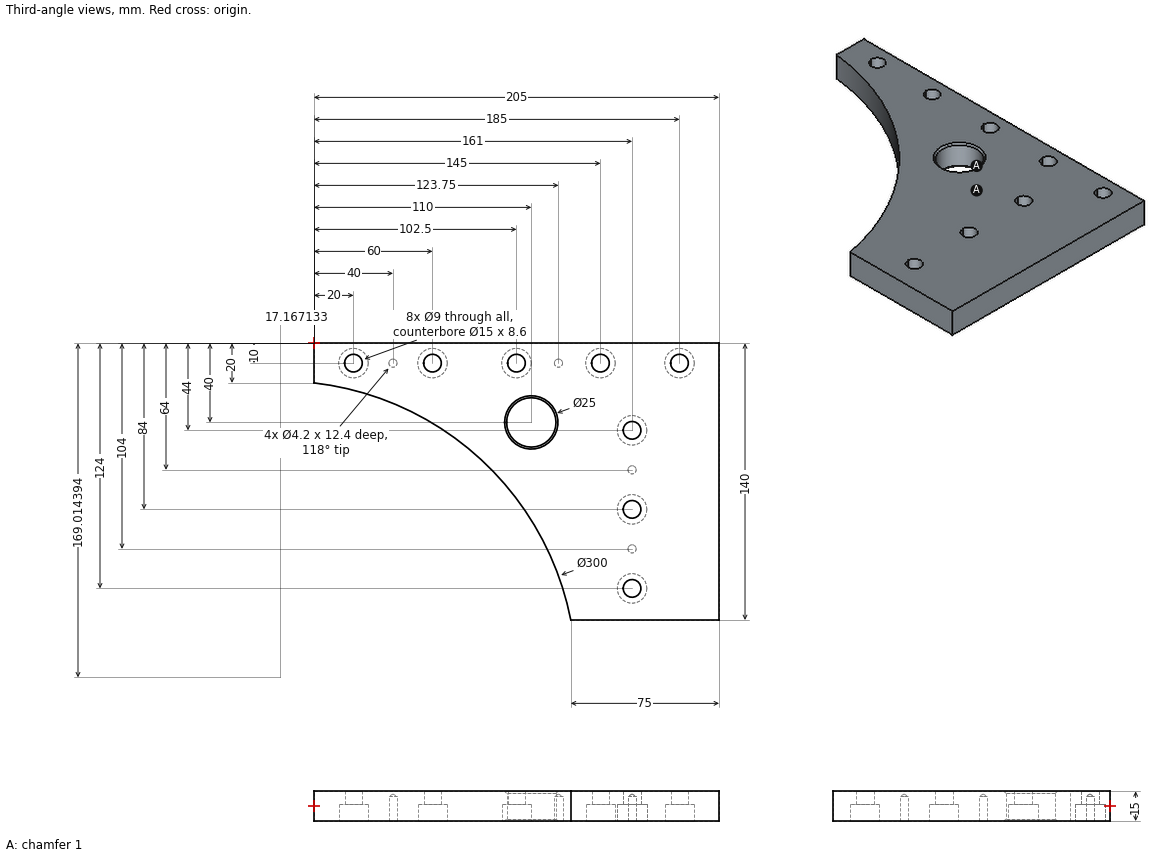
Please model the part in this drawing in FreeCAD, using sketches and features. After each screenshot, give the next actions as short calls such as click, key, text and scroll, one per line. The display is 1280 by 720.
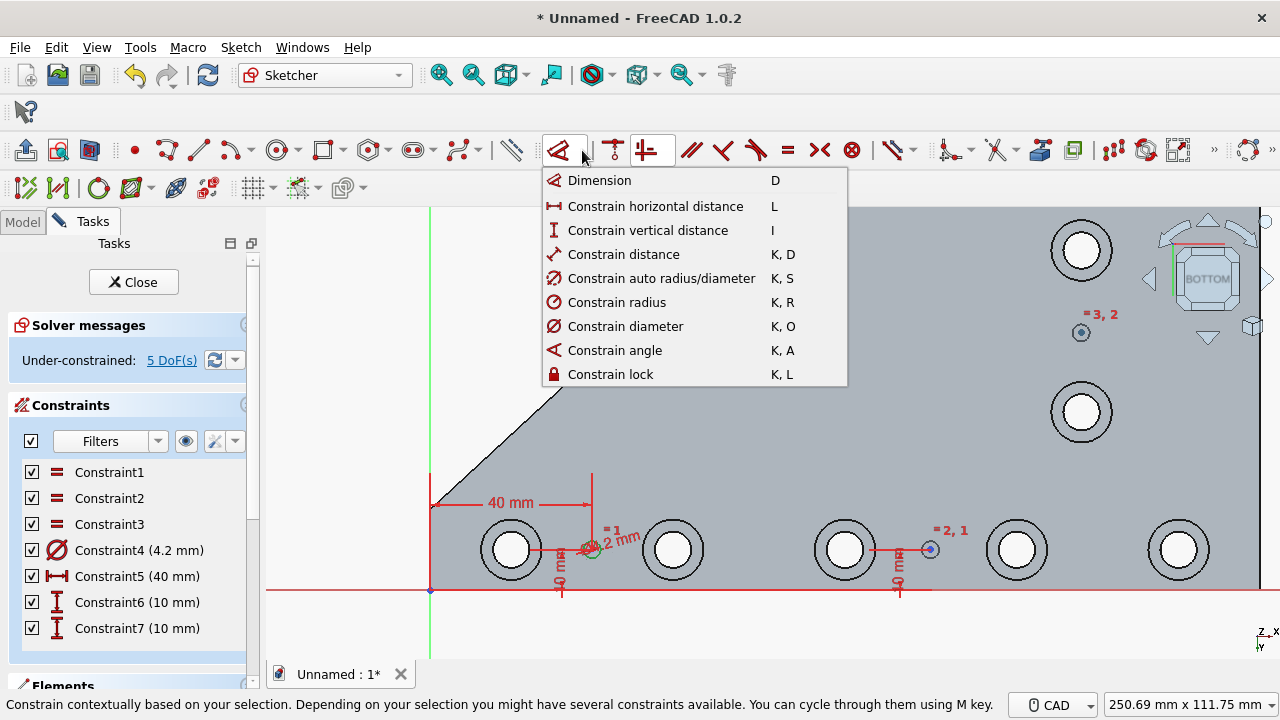
click(695, 230)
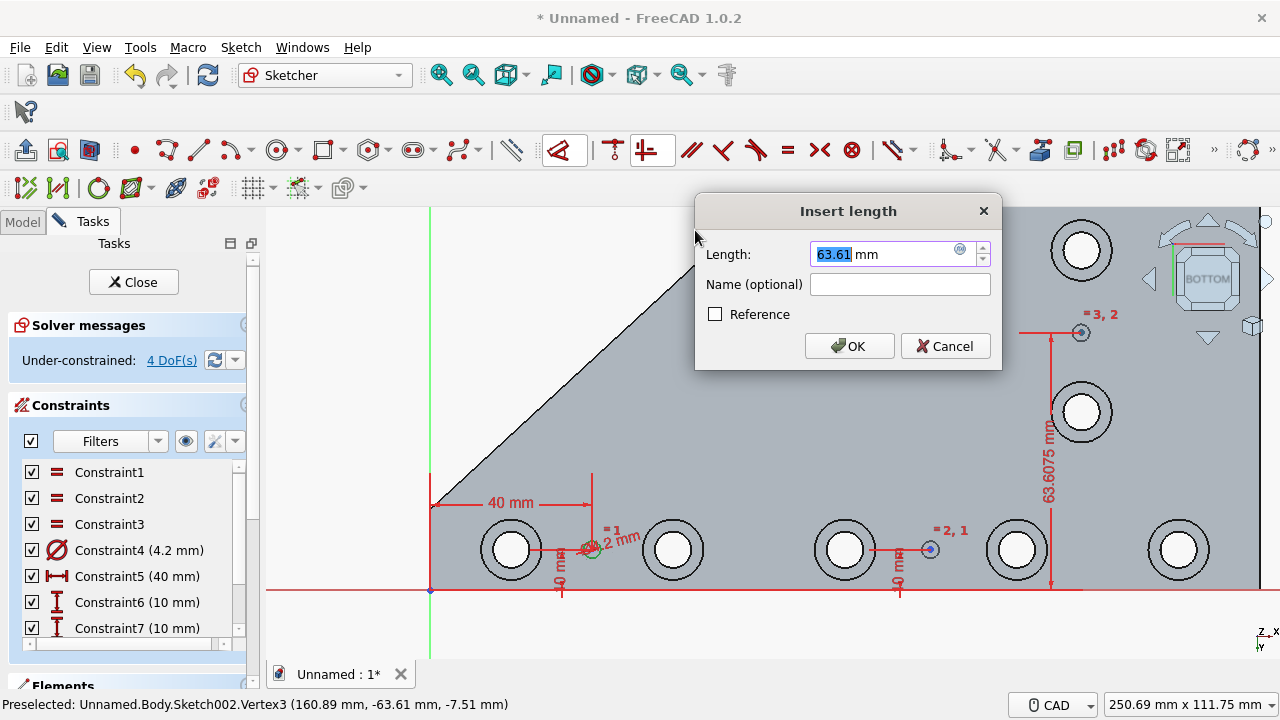
text(64)
key(Return)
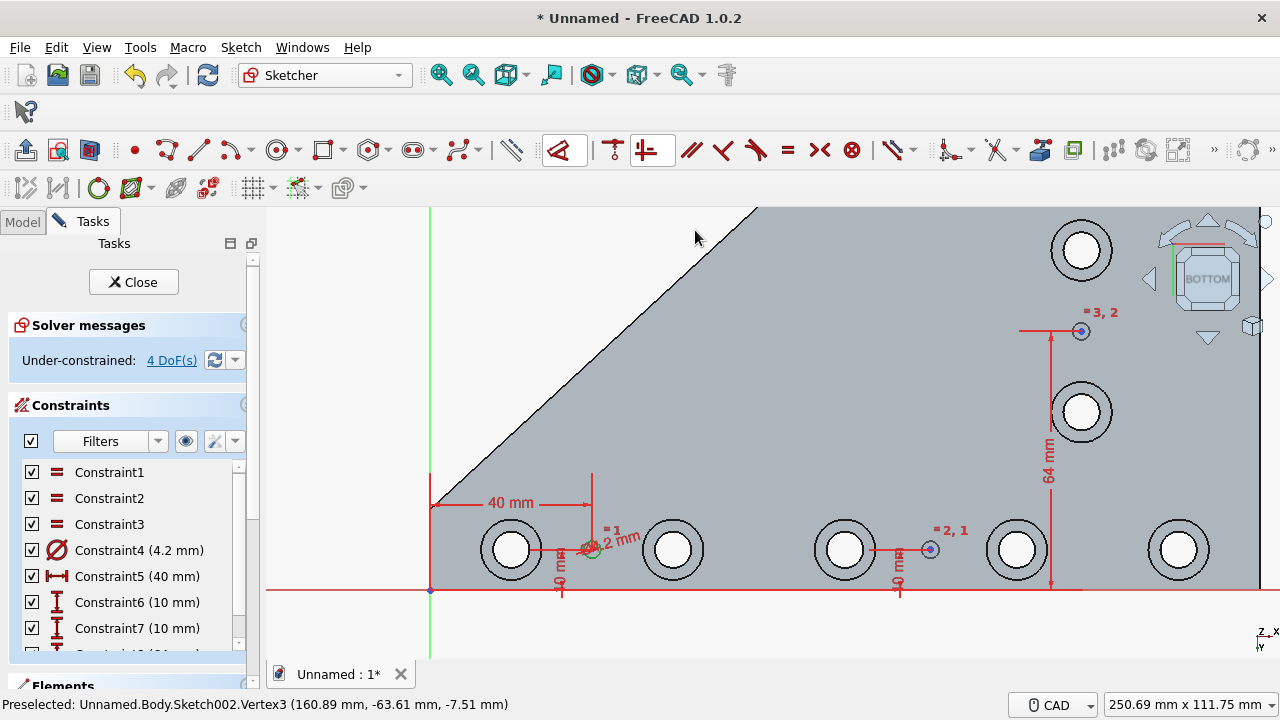
click(1081, 331)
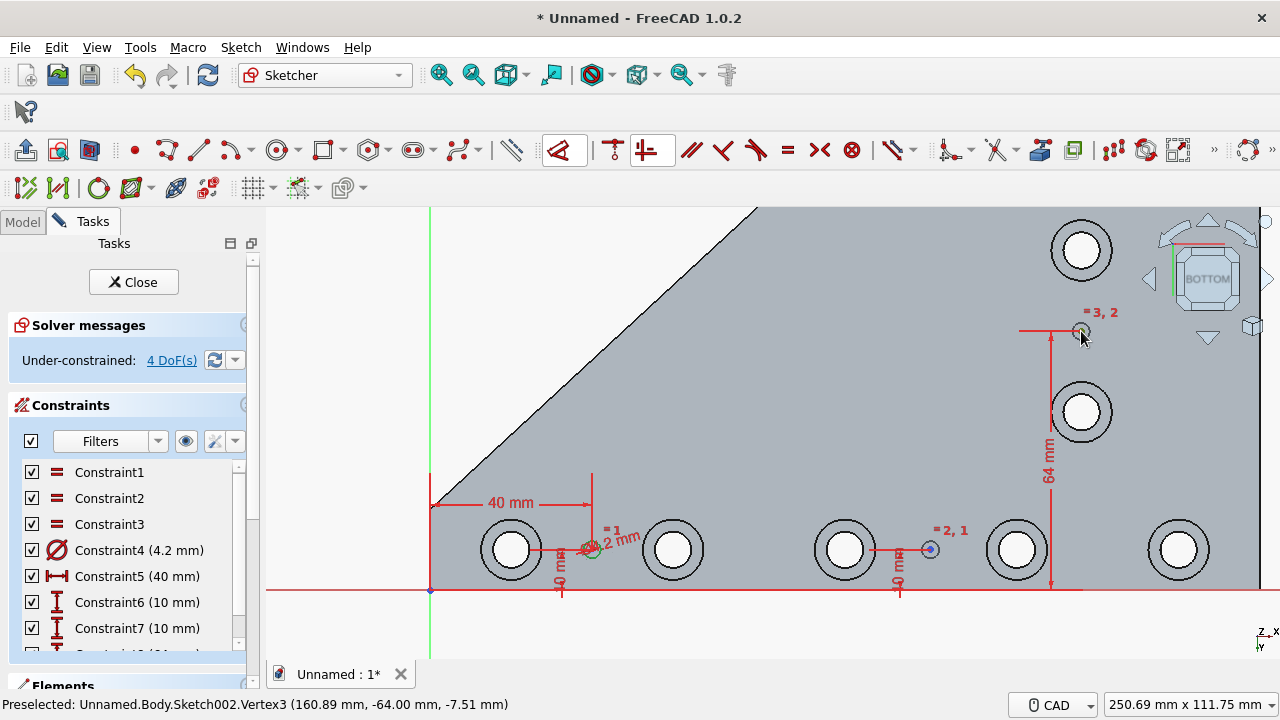
key(l)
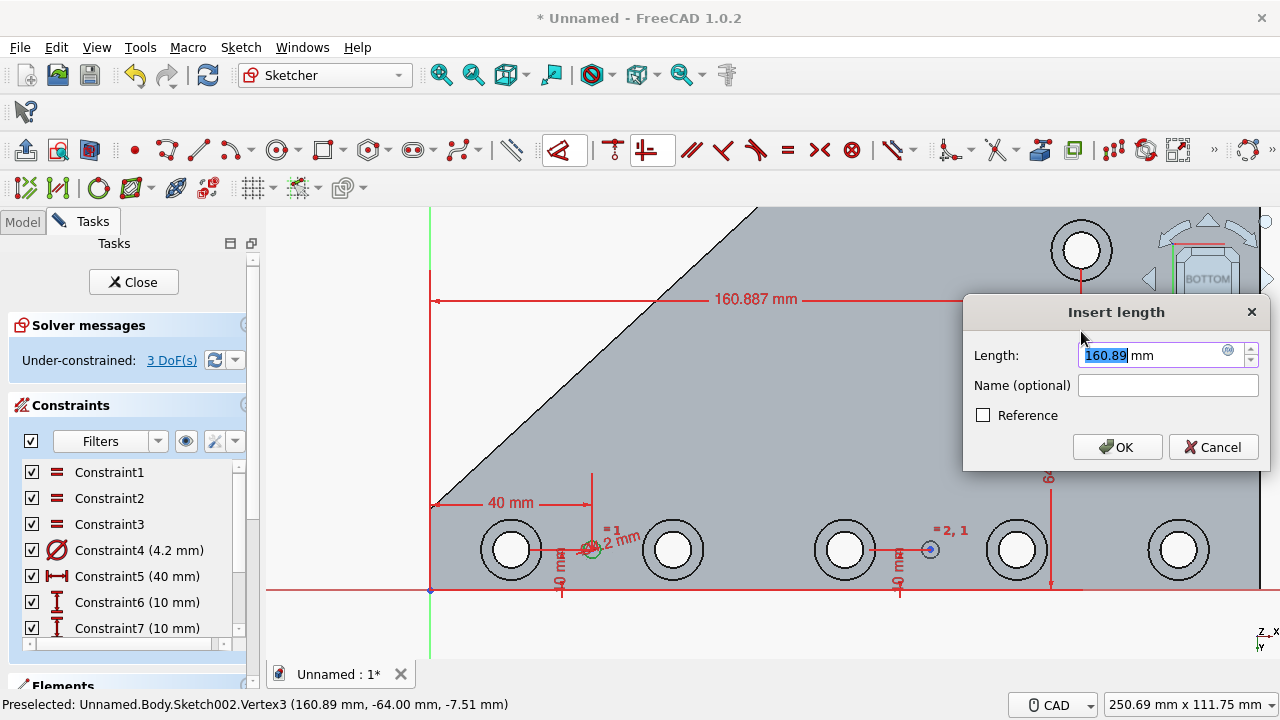
text(161)
key(Return)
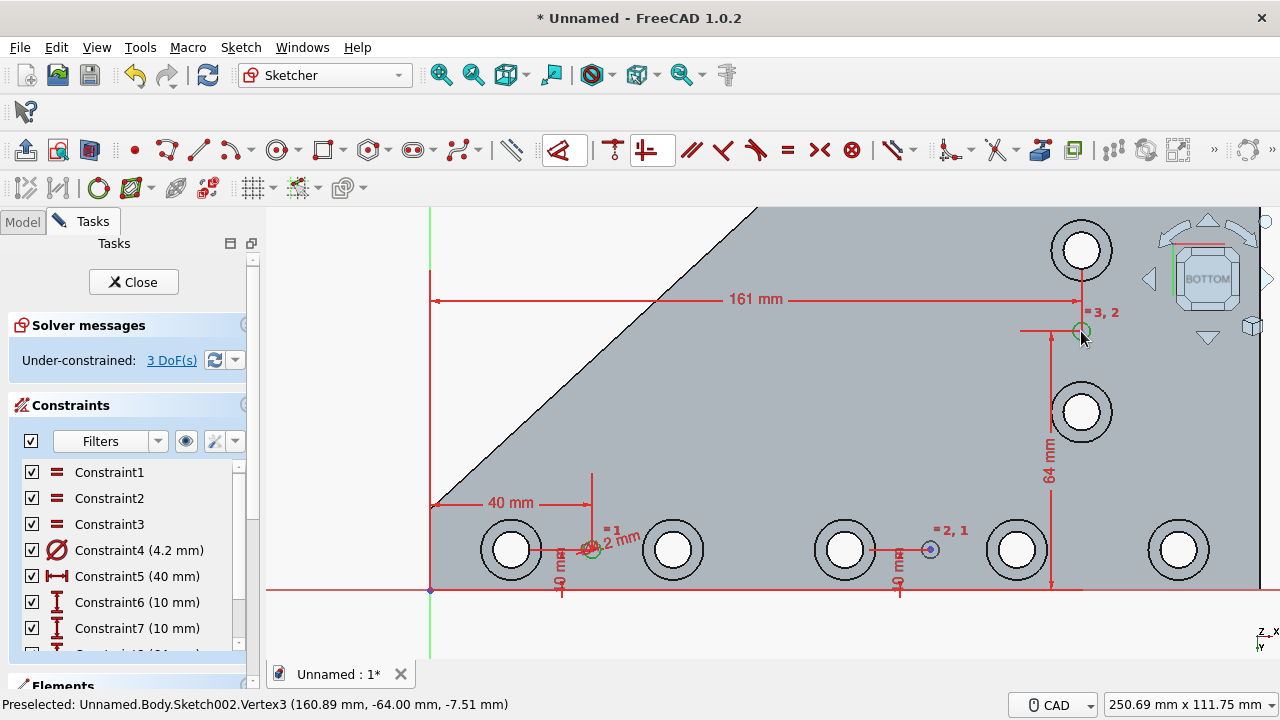
scroll(591, 550, down, 2)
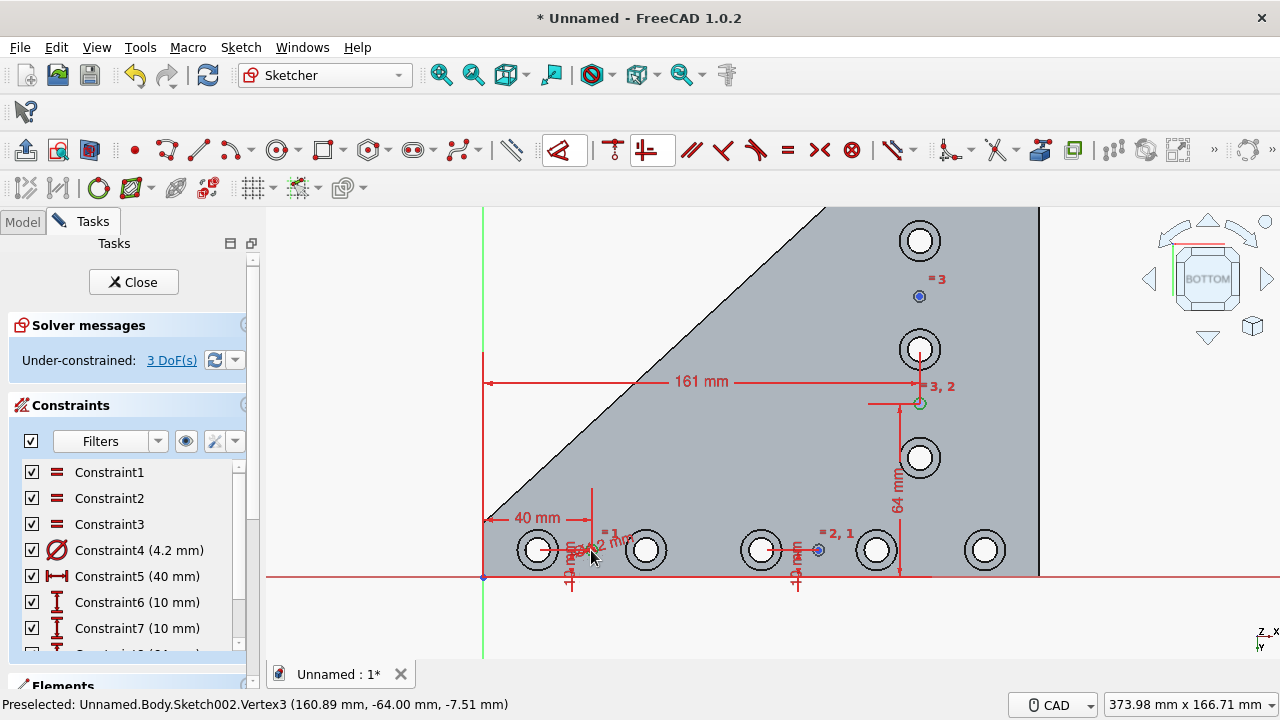
click(920, 297)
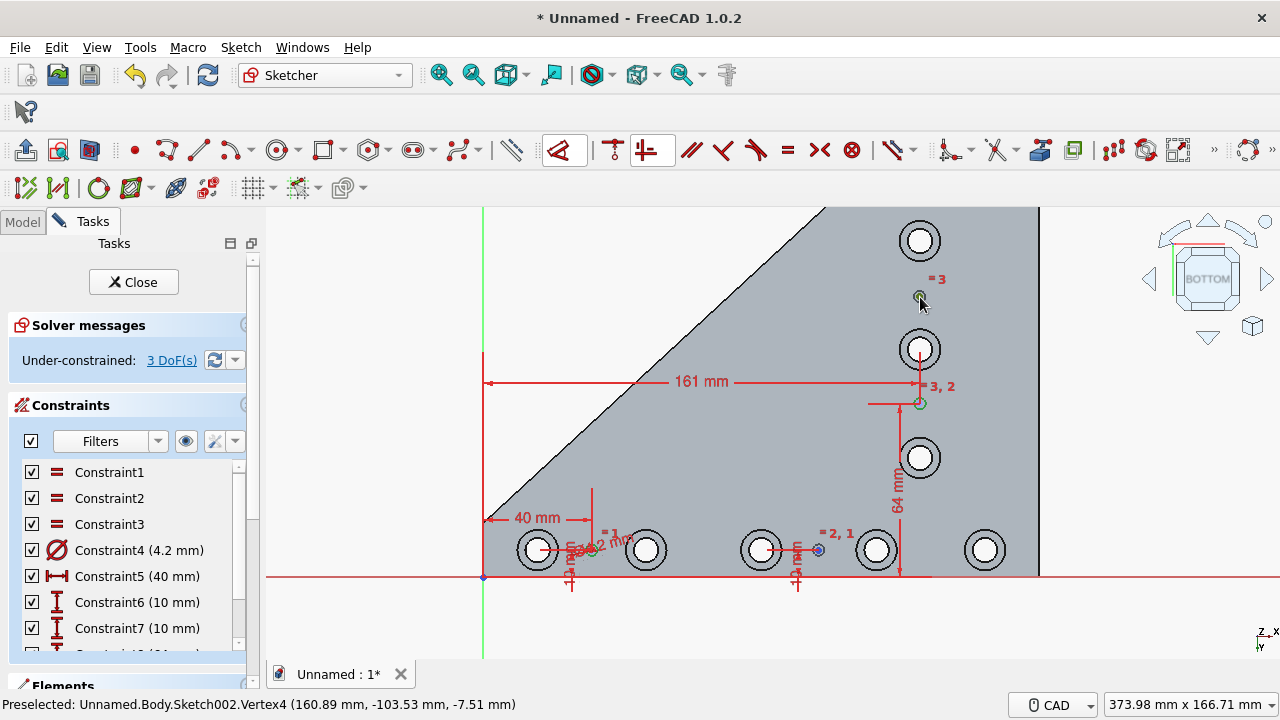
key(l)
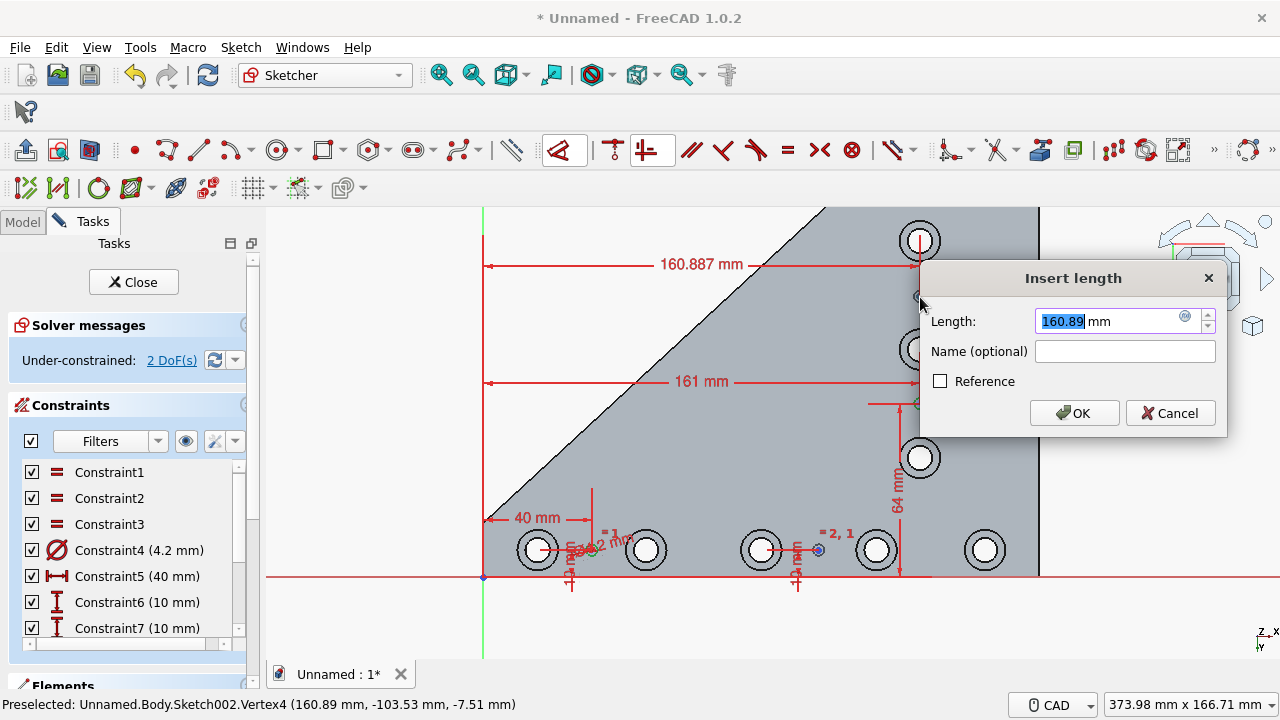
text(161)
key(Return)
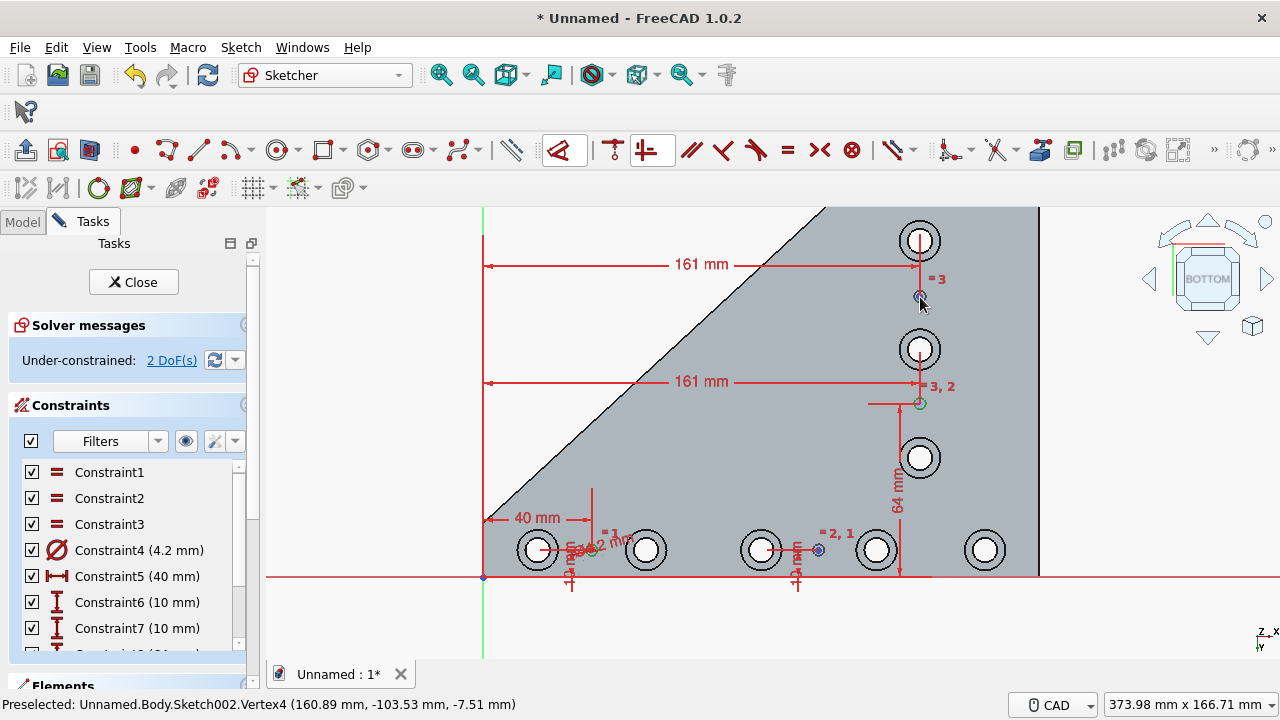
click(920, 297)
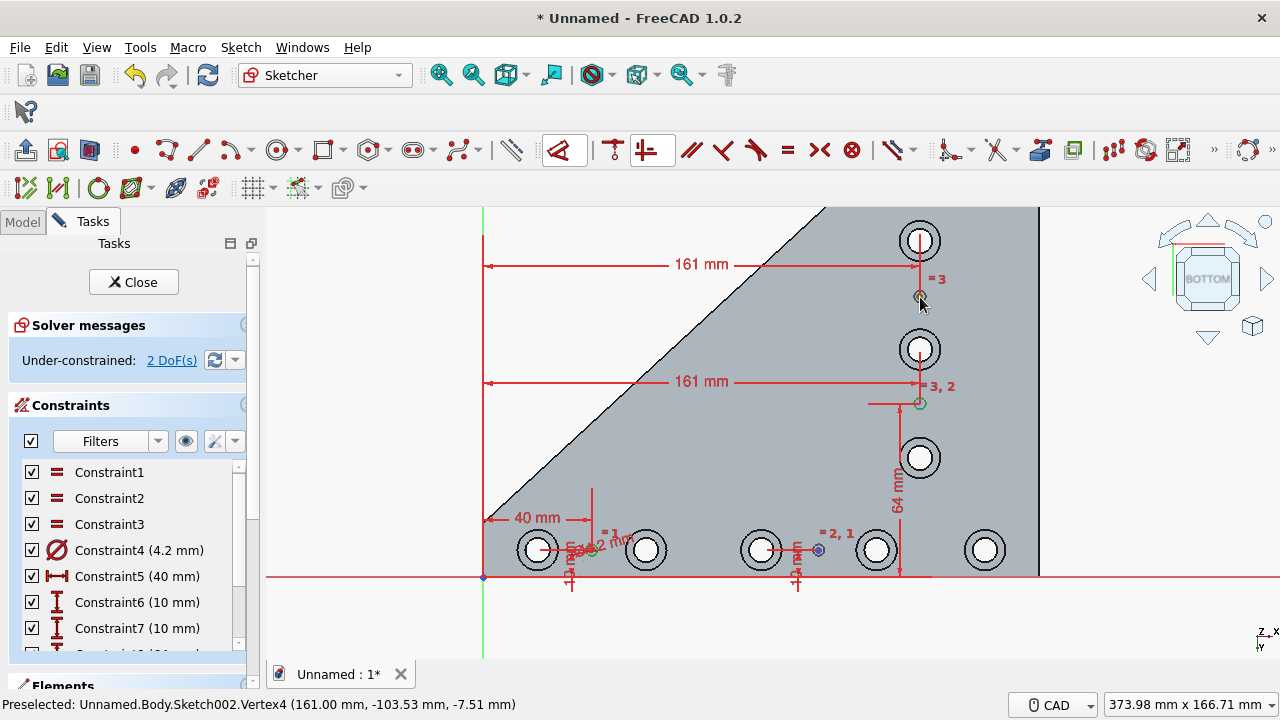
click(582, 150)